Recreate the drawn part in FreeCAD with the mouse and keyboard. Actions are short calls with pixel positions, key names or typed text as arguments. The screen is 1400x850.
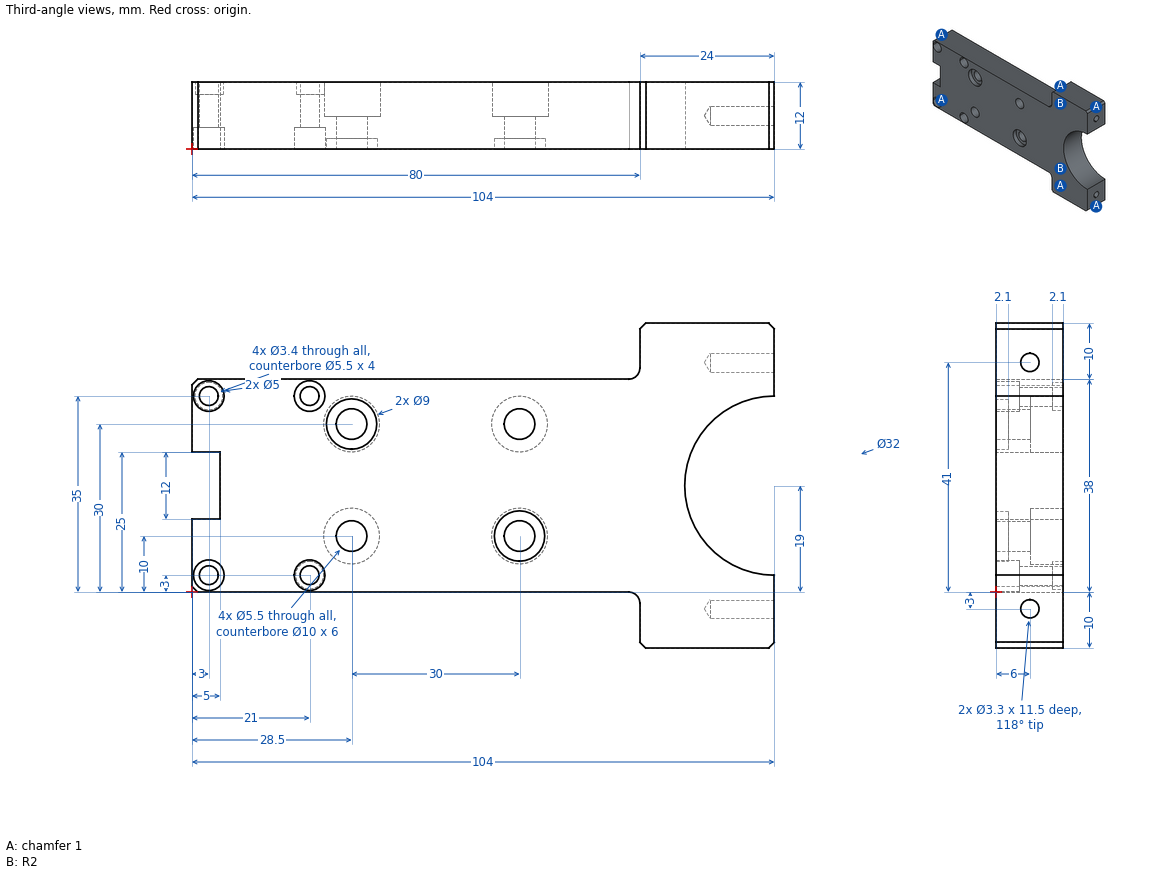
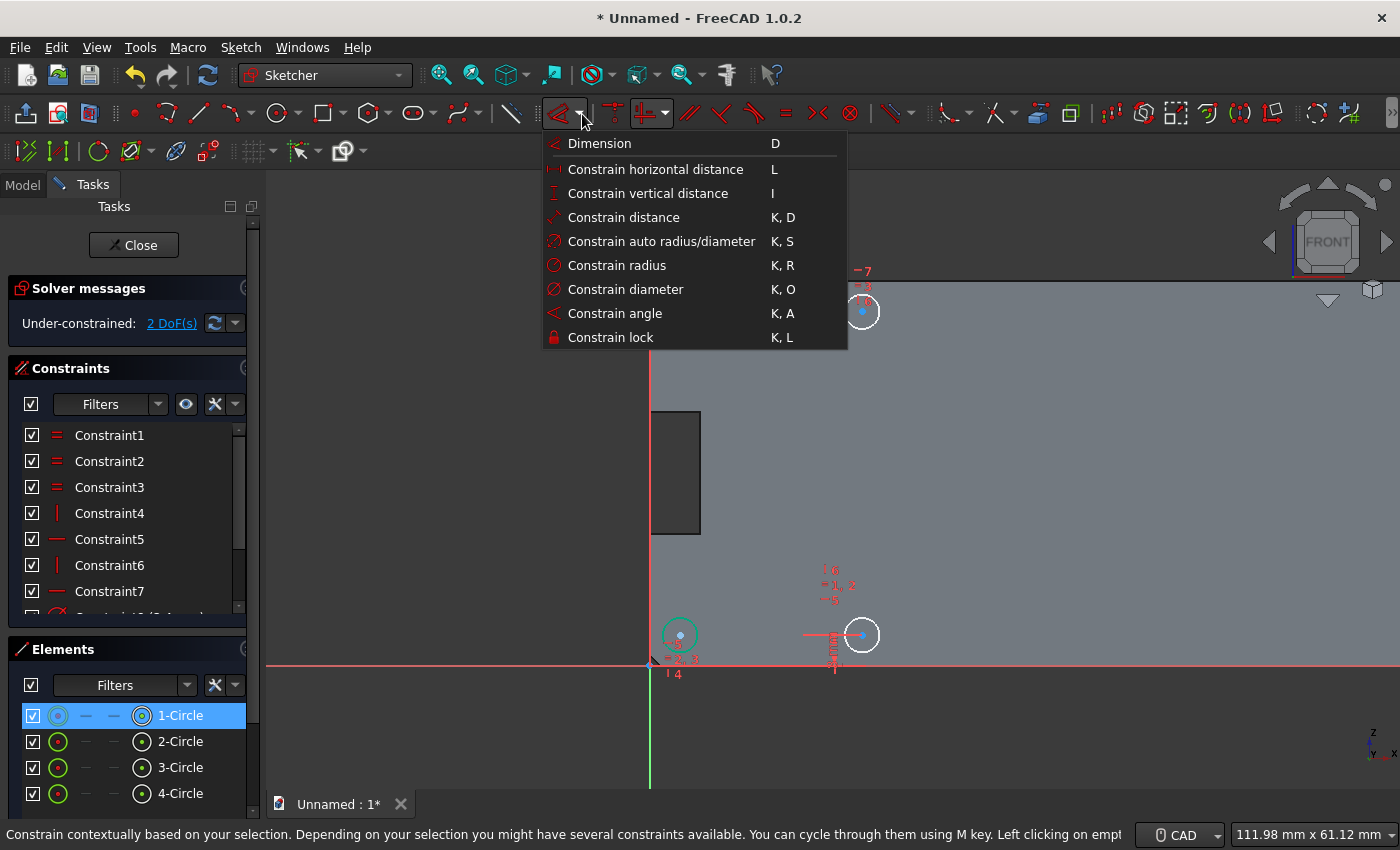
click(695, 193)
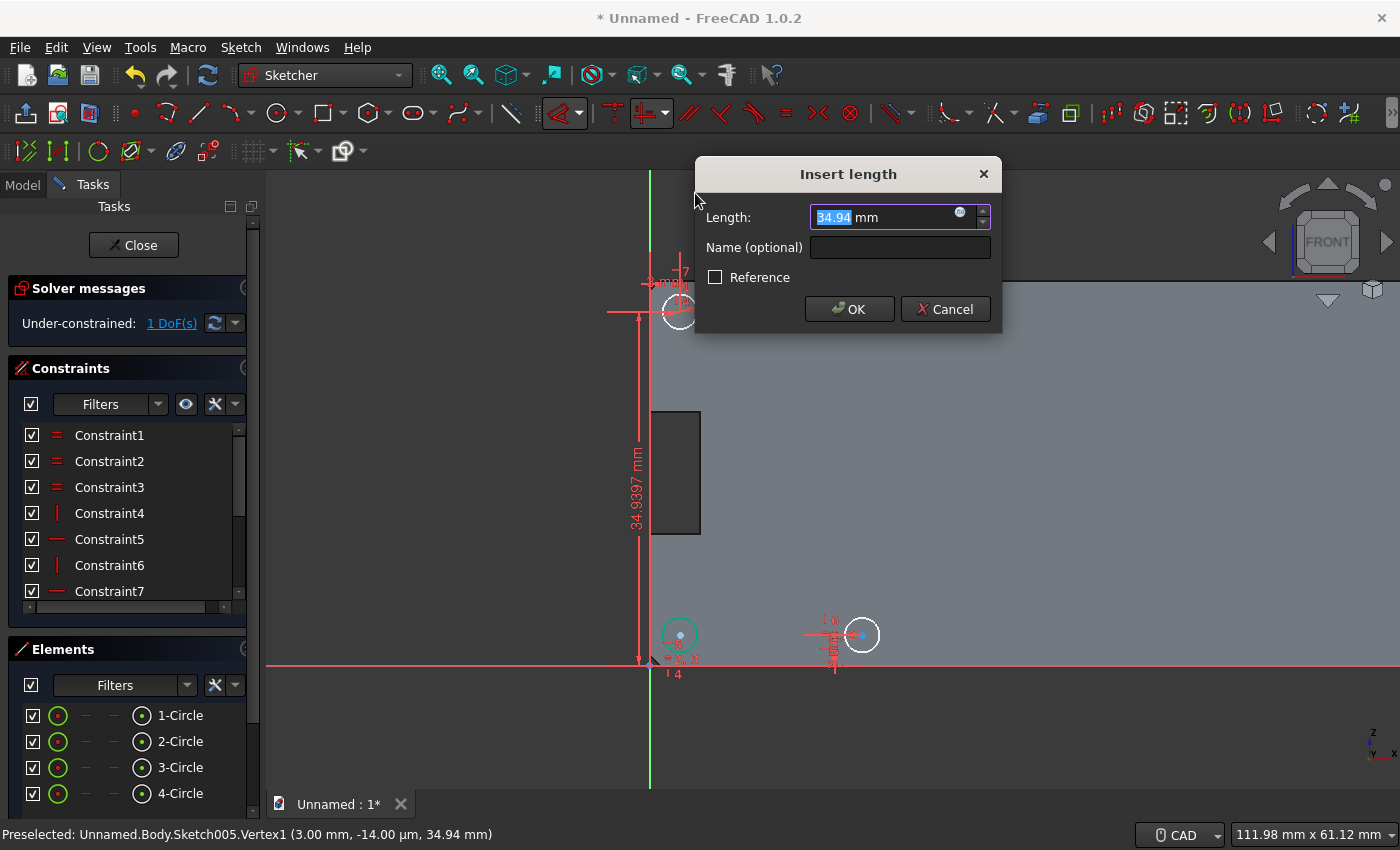
text(35)
key(Return)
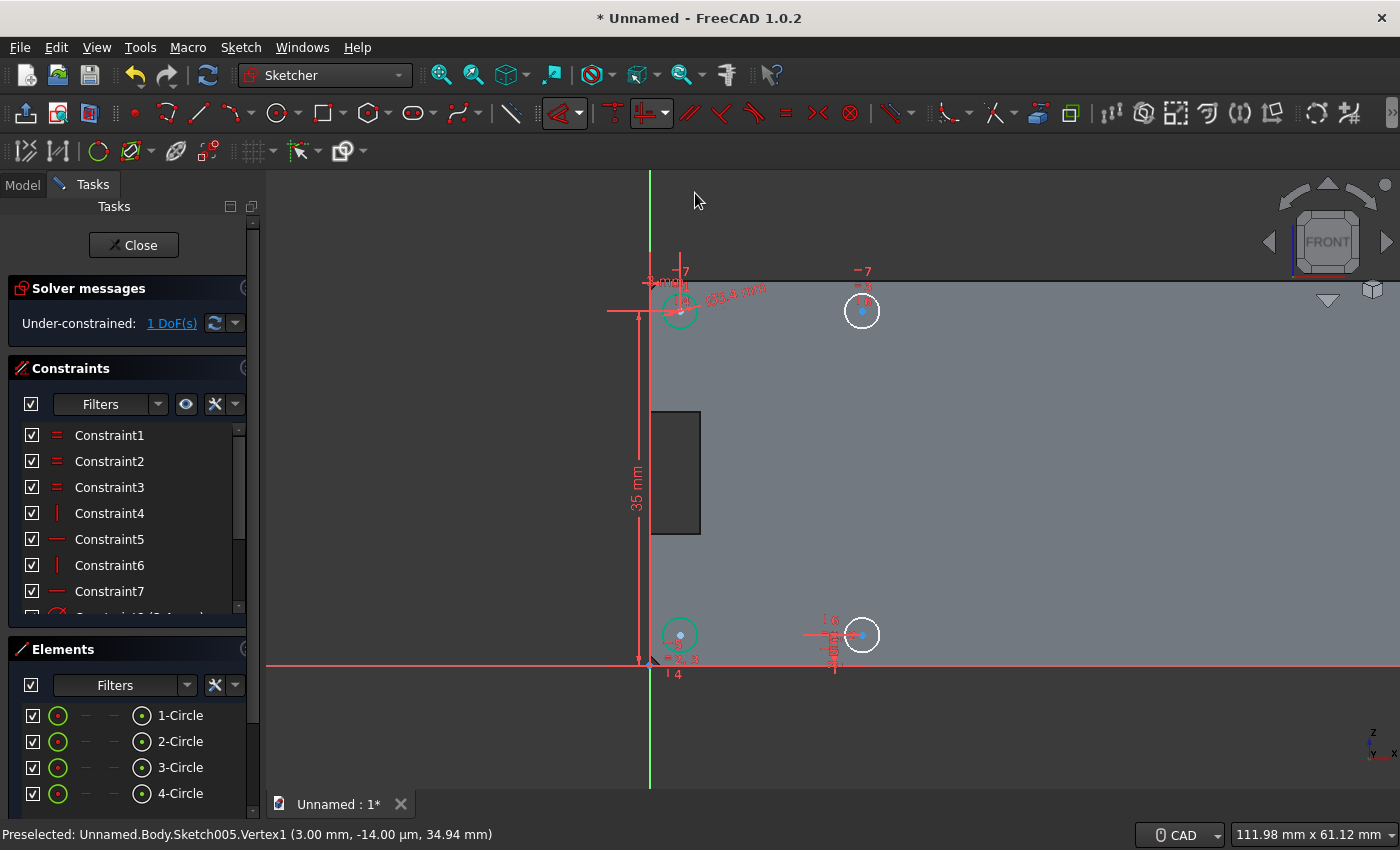
click(862, 635)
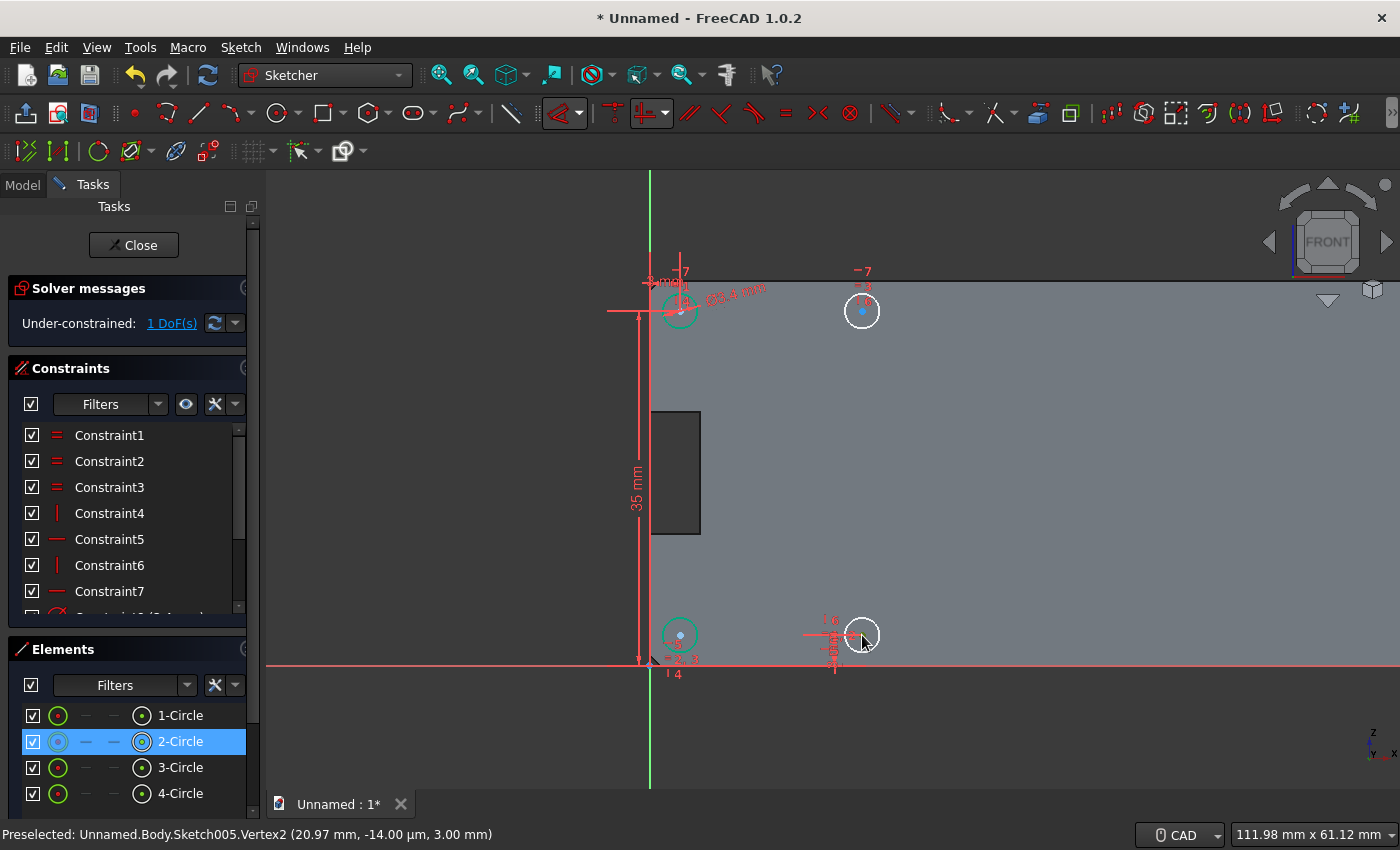
click(582, 114)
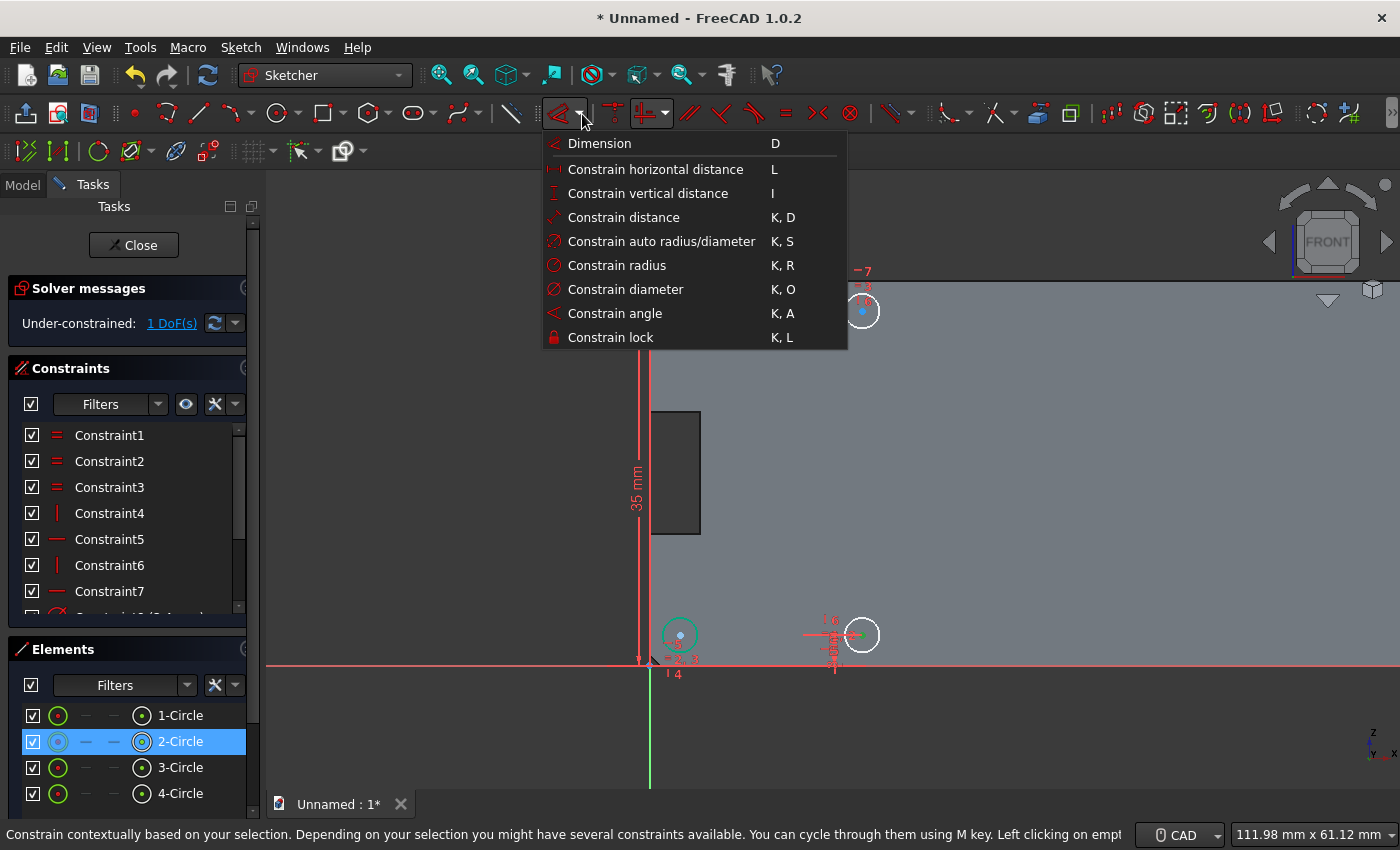
click(695, 169)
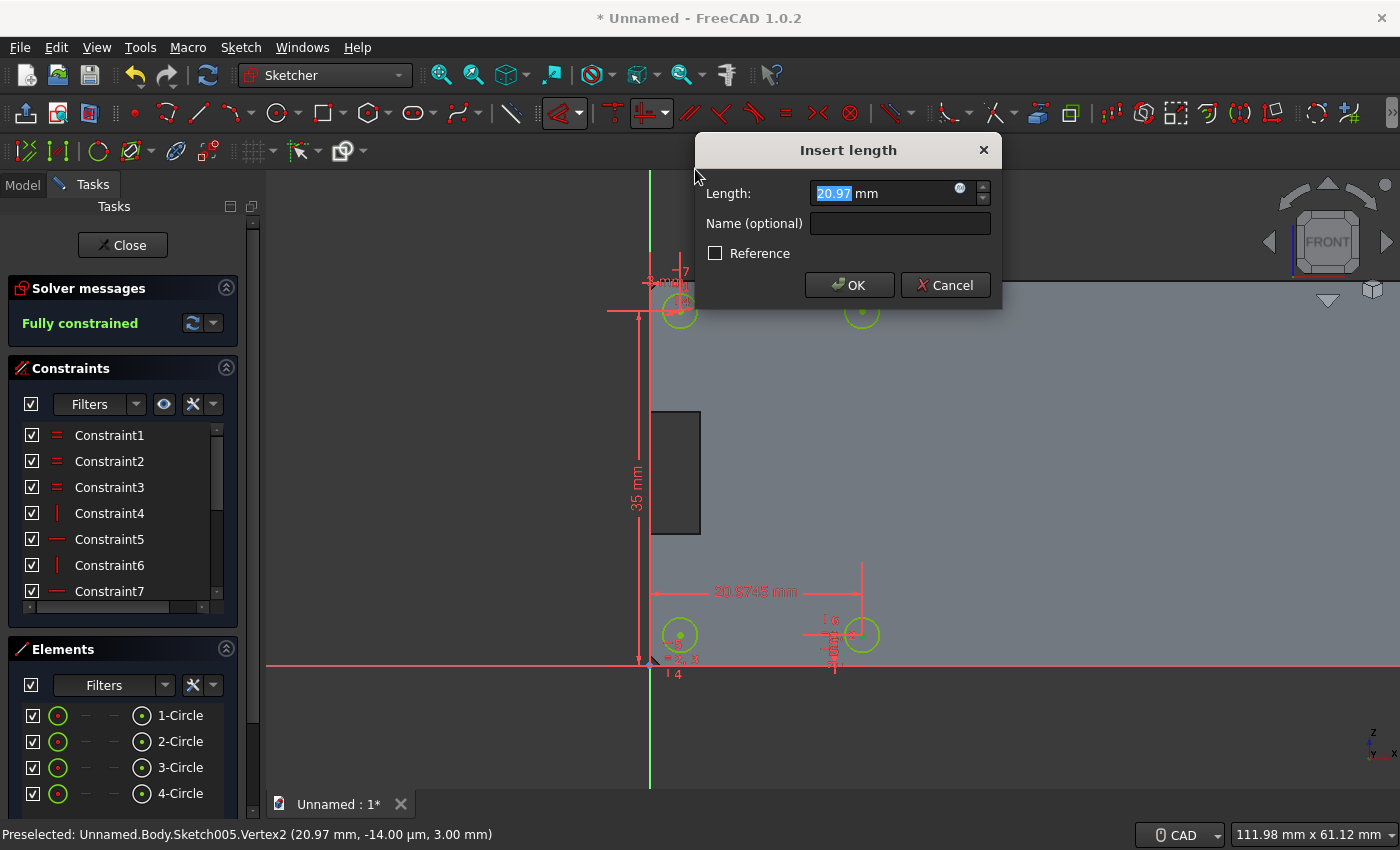
text(21)
key(Return)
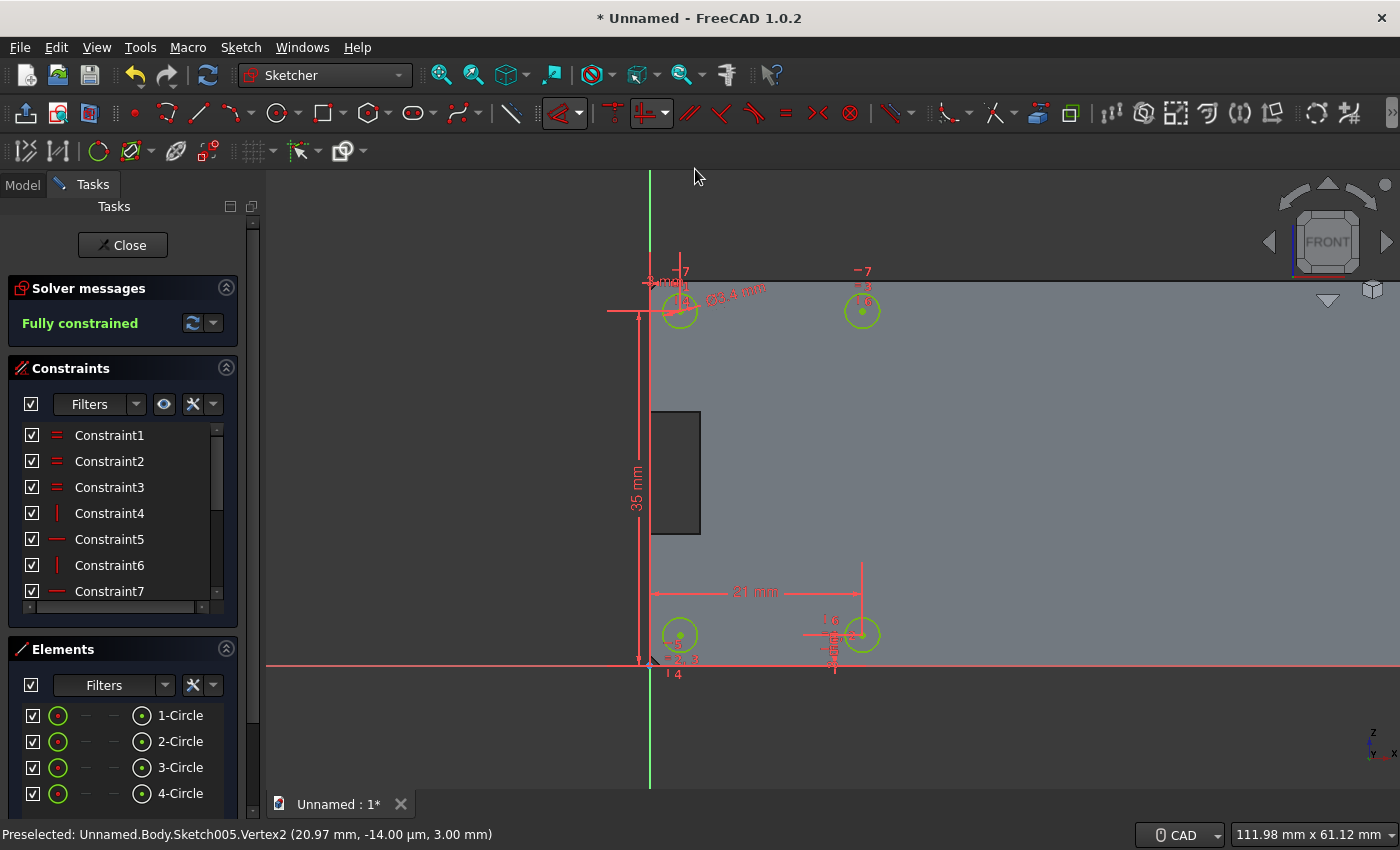
click(123, 245)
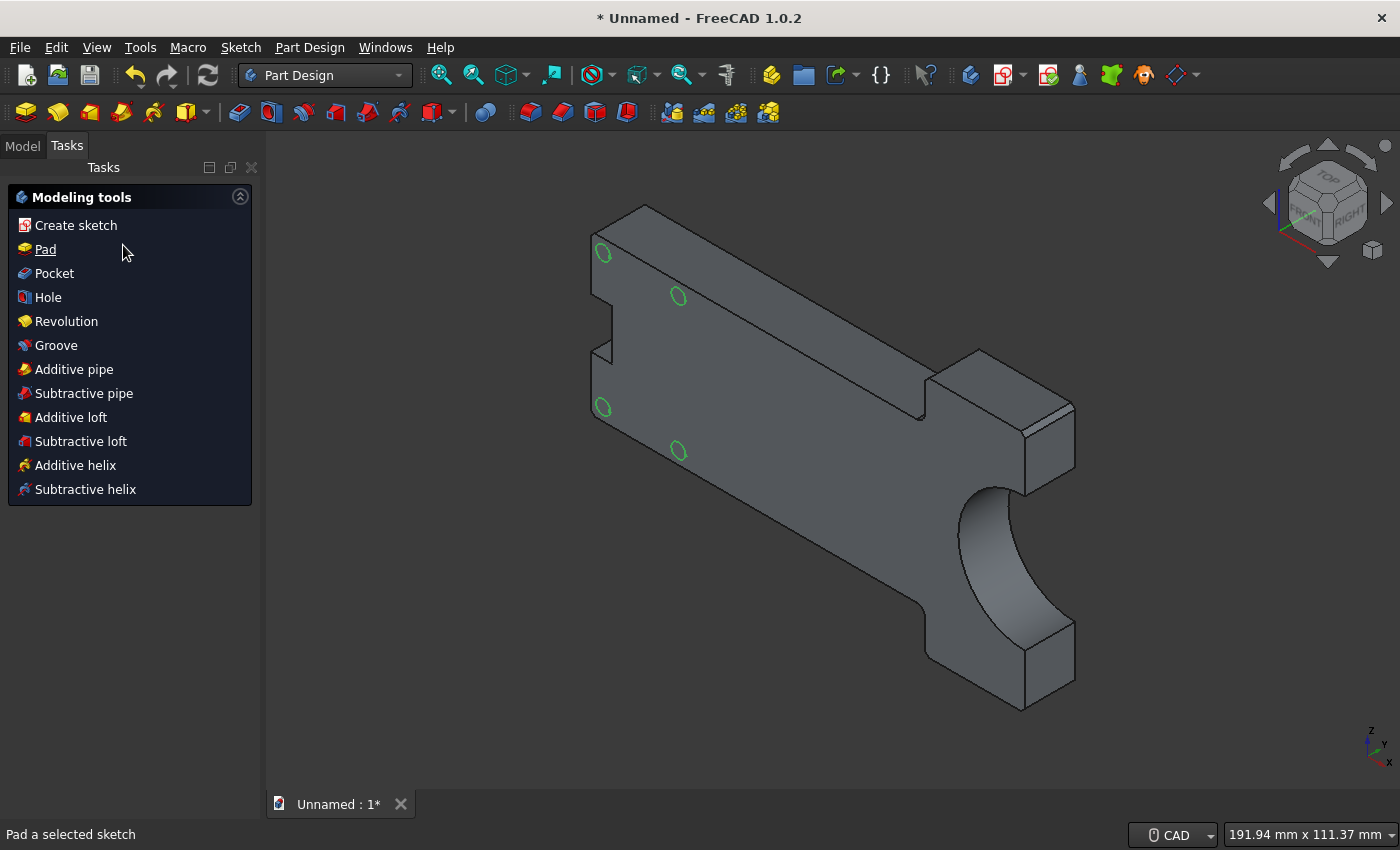
click(272, 112)